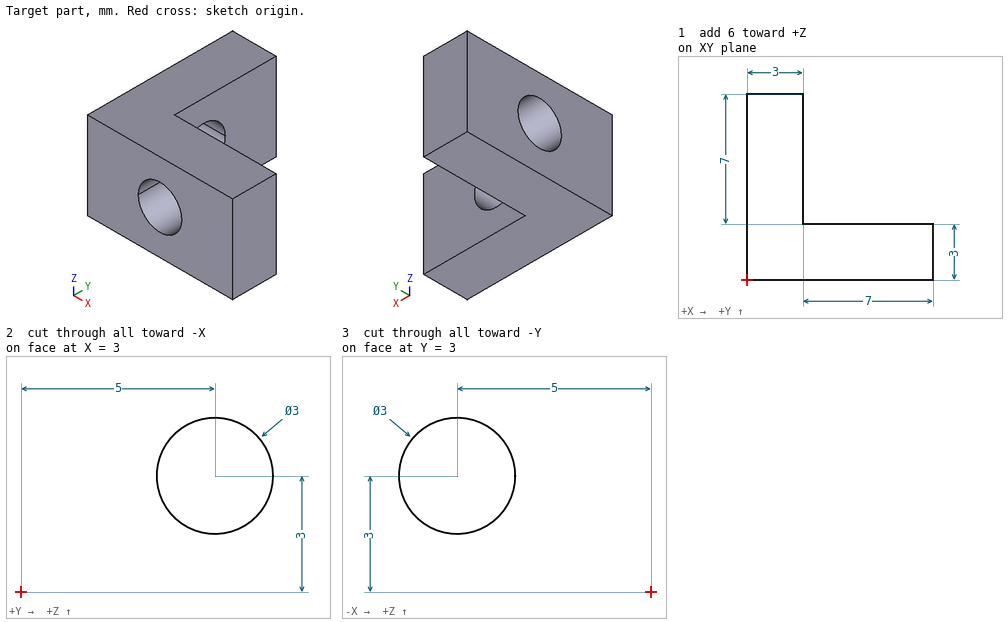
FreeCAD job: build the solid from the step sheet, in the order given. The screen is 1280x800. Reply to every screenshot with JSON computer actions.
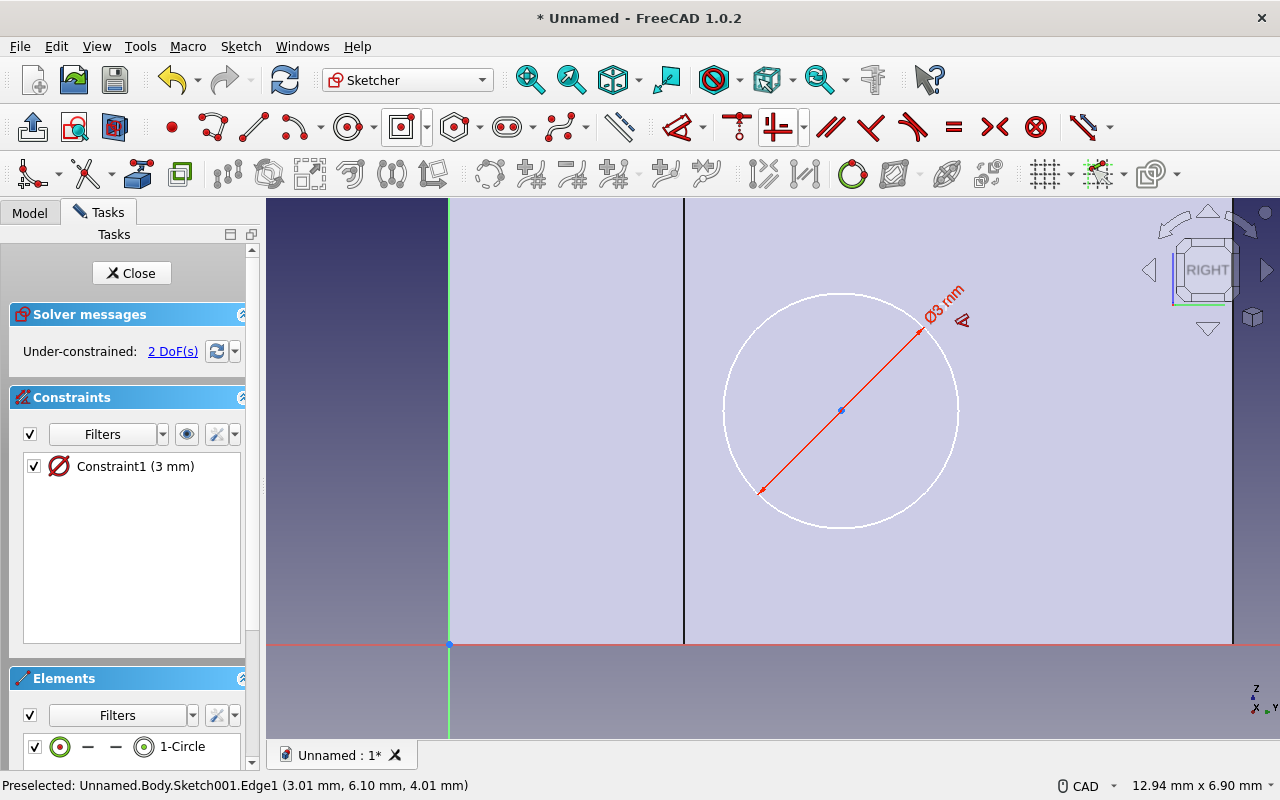
{"action": "left_click", "coordinate": [841, 411]}
{"action": "left_click", "coordinate": [645, 679]}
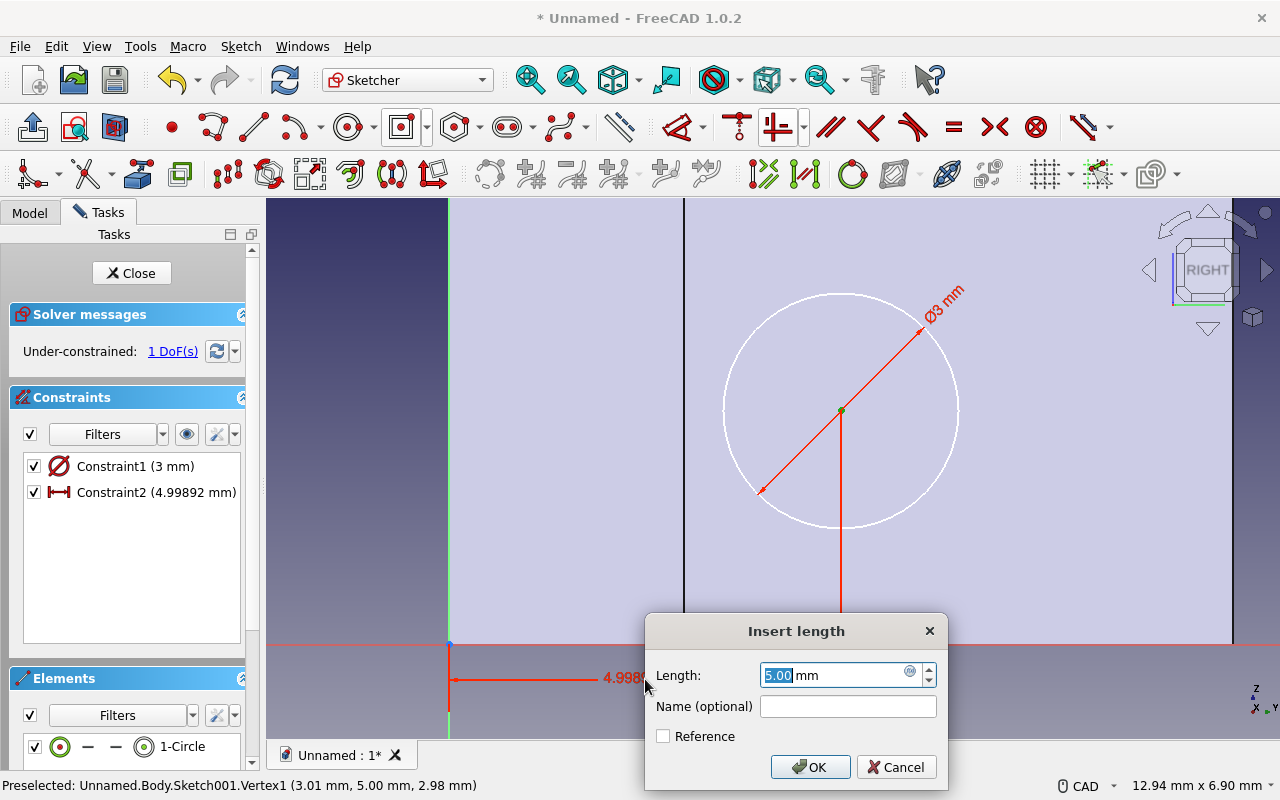
{"action": "type", "text": "5"}
{"action": "key", "text": "Return"}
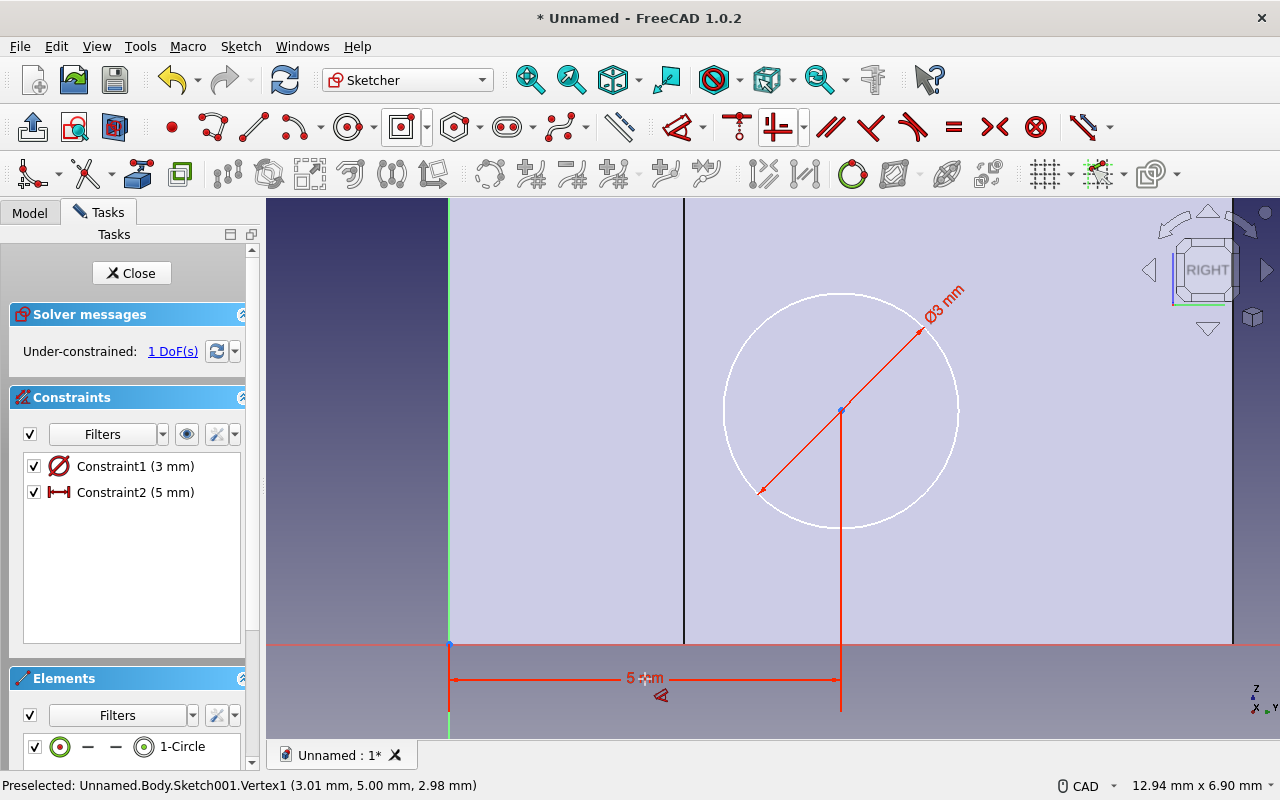
{"action": "left_click", "coordinate": [841, 411]}
{"action": "left_click", "coordinate": [415, 528]}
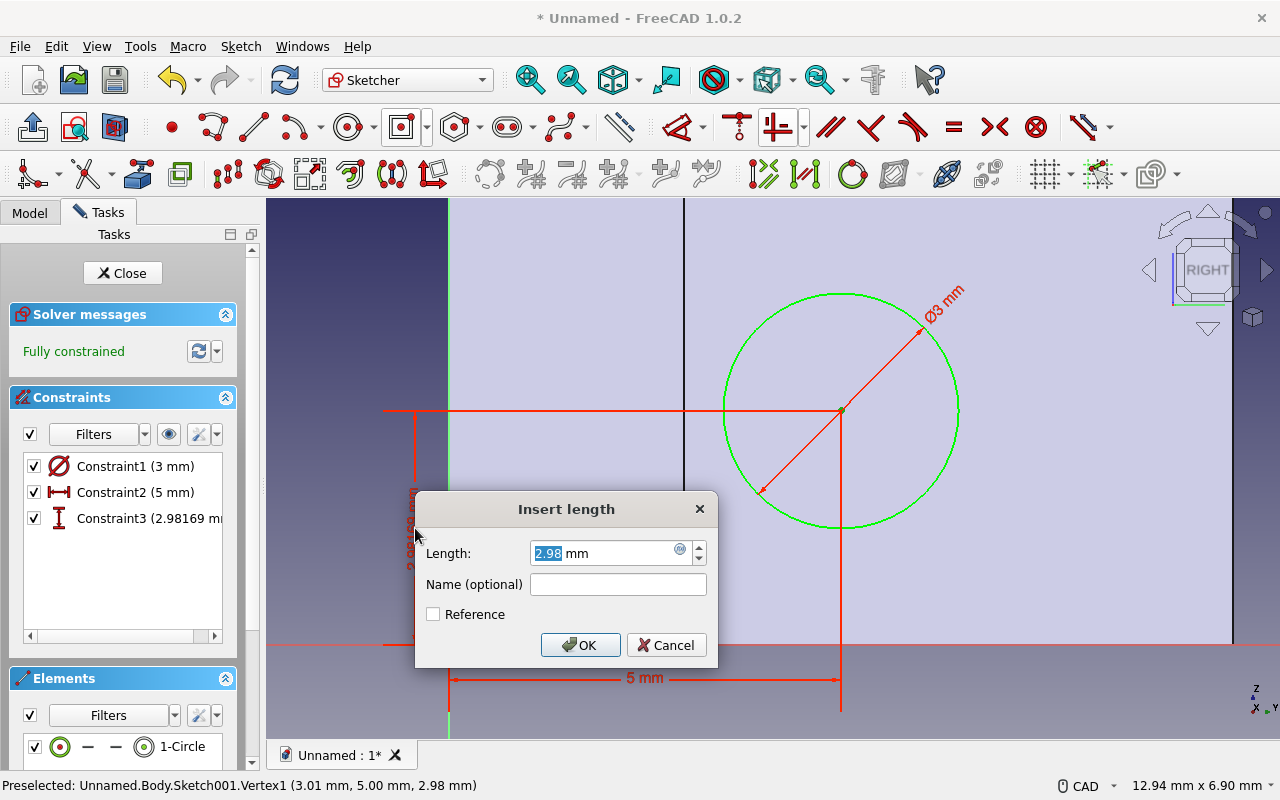
{"action": "type", "text": "3"}
{"action": "key", "text": "Return"}
{"action": "key", "text": "Escape"}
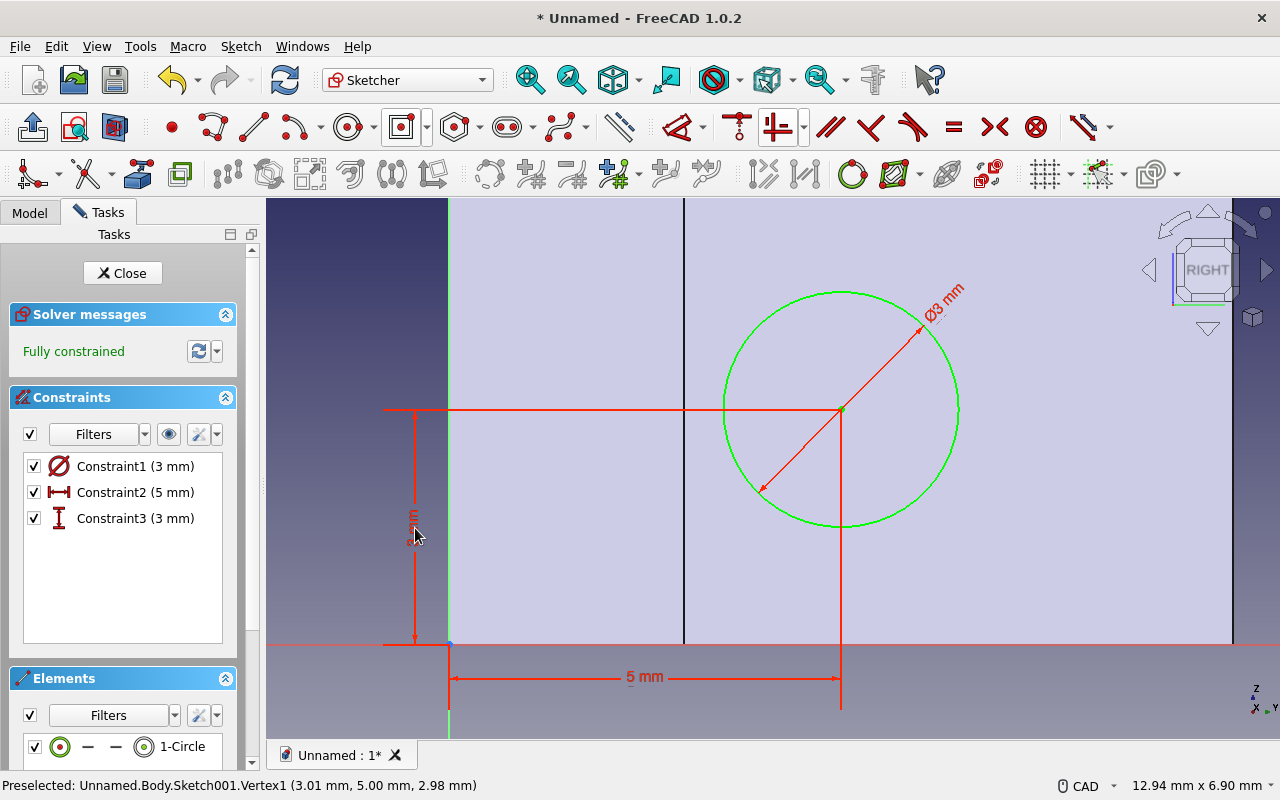
{"action": "left_click", "coordinate": [123, 273]}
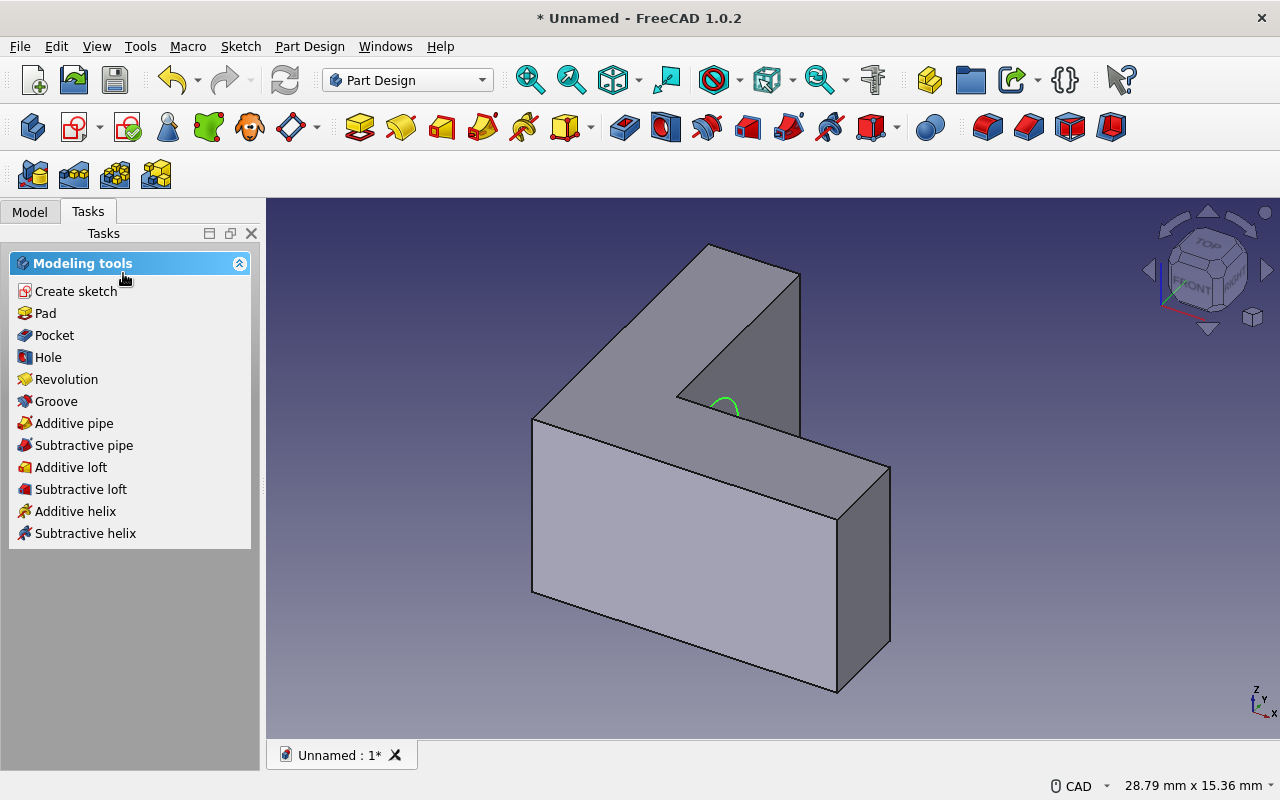
{"action": "left_click", "coordinate": [625, 128]}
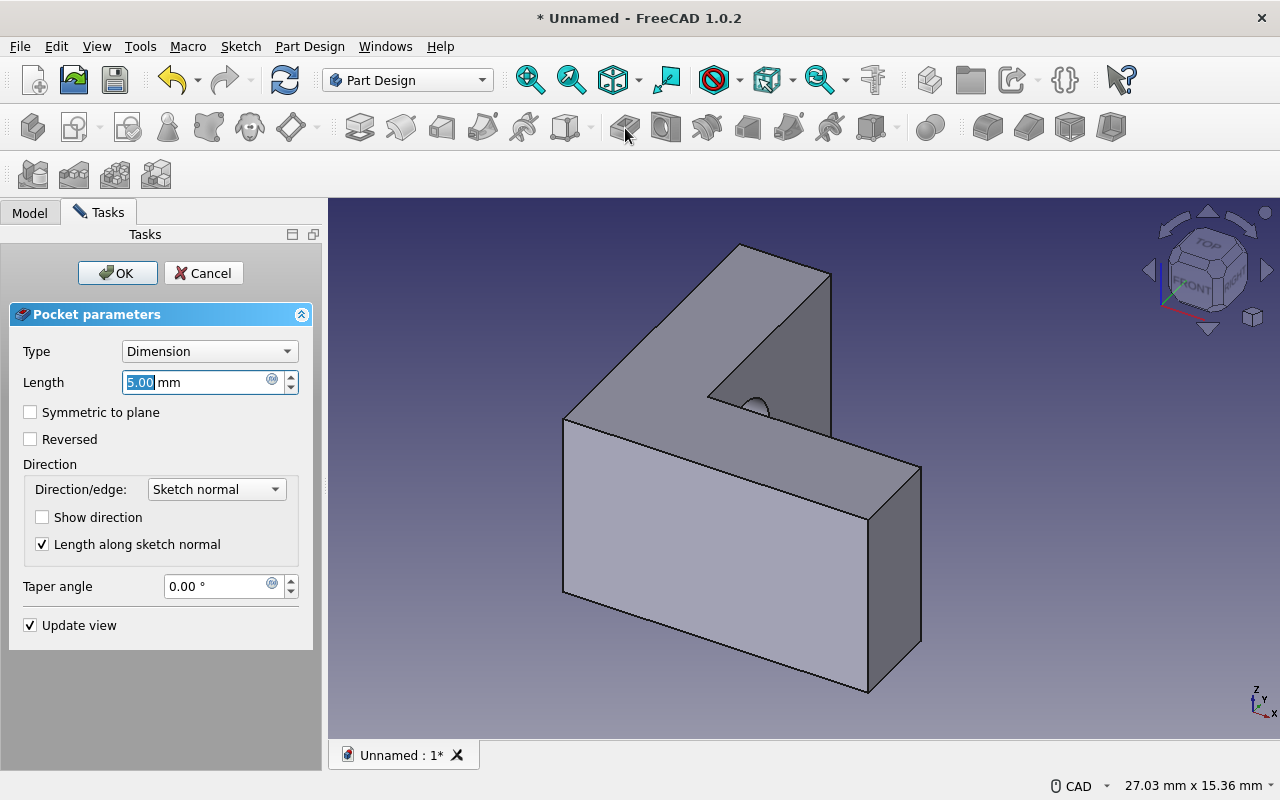
{"action": "left_click", "coordinate": [210, 352]}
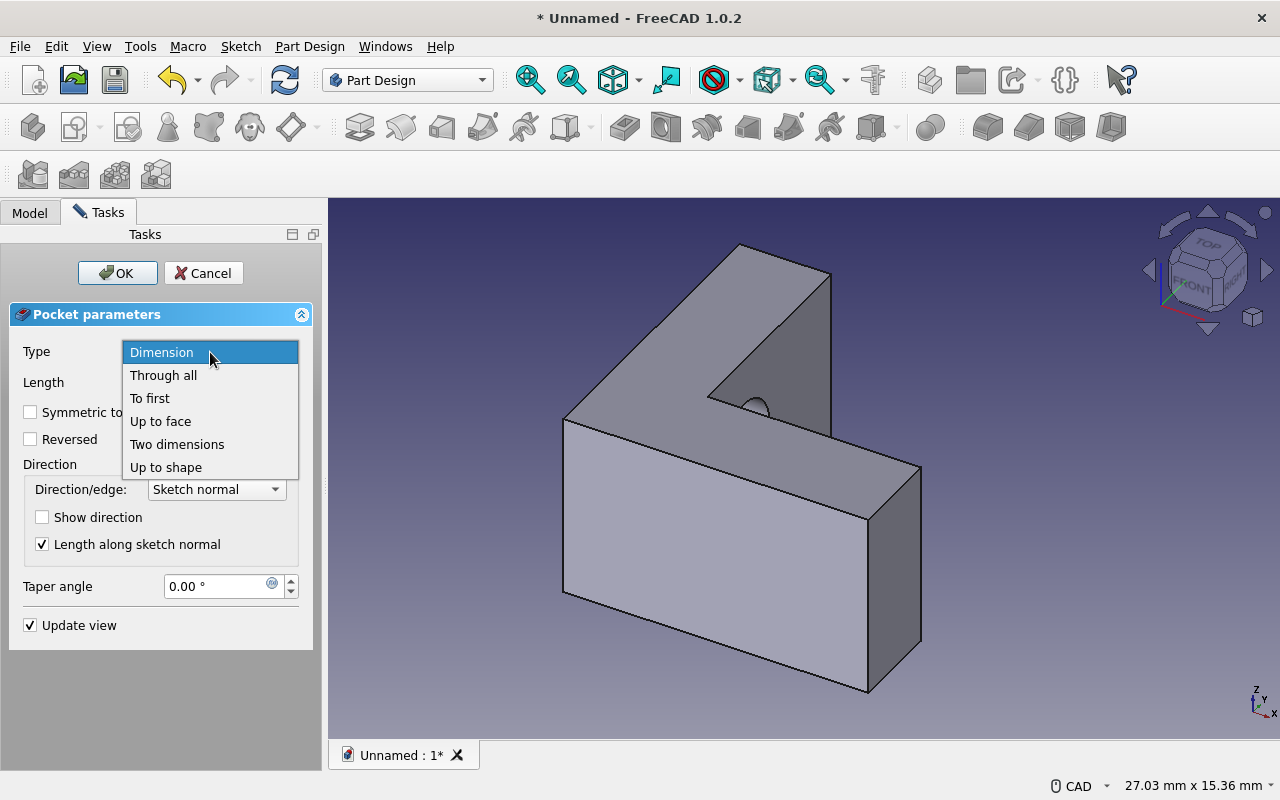
{"action": "left_click", "coordinate": [208, 376]}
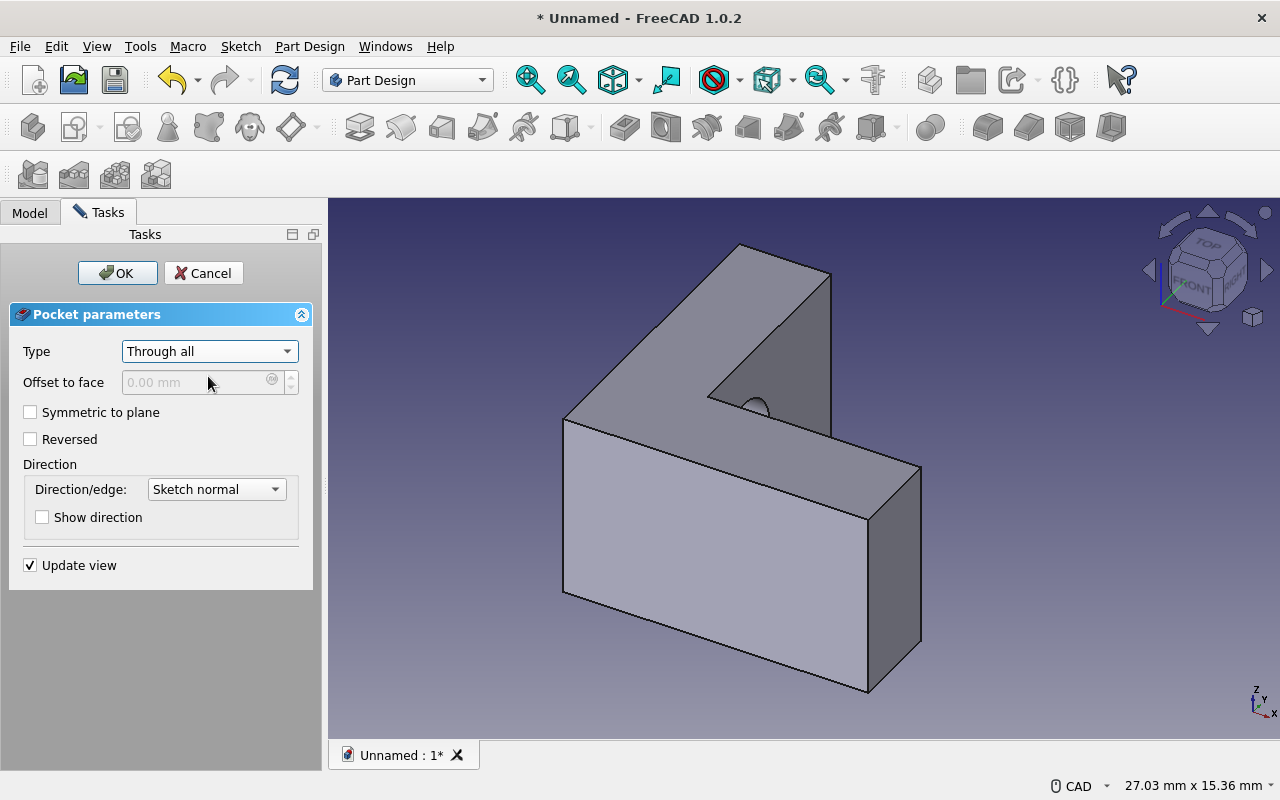
{"action": "left_click", "coordinate": [118, 273]}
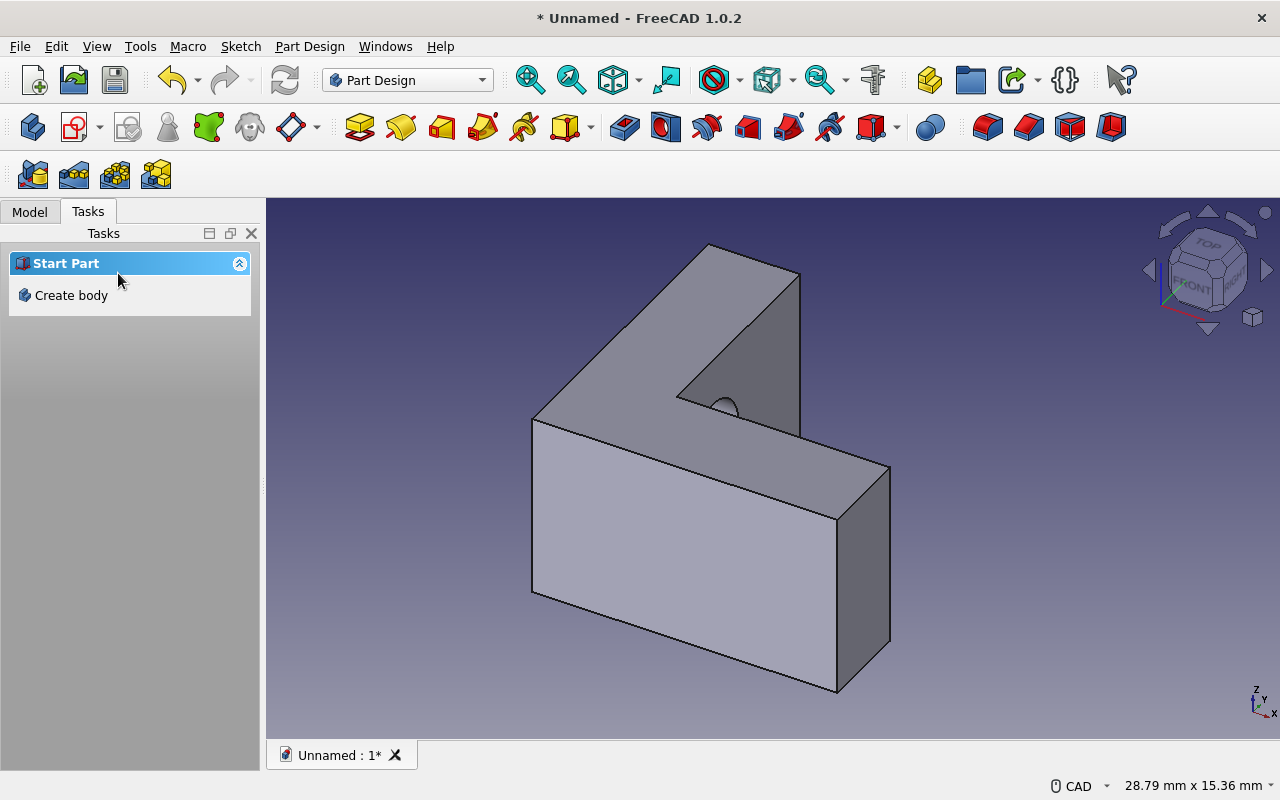
{"action": "key", "text": "4"}